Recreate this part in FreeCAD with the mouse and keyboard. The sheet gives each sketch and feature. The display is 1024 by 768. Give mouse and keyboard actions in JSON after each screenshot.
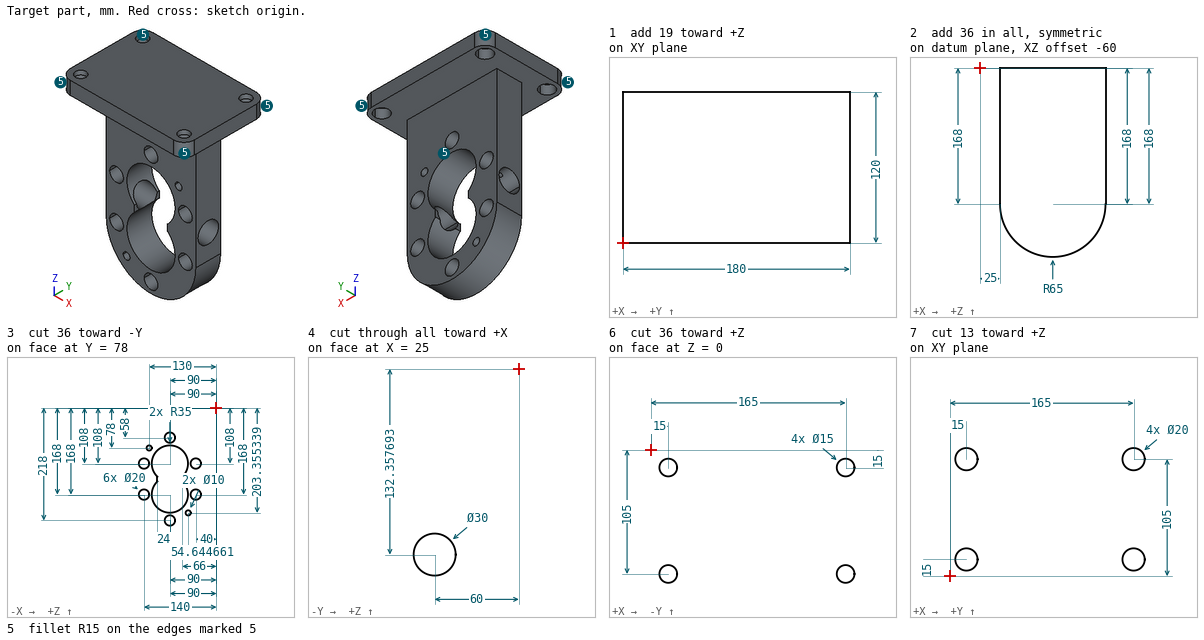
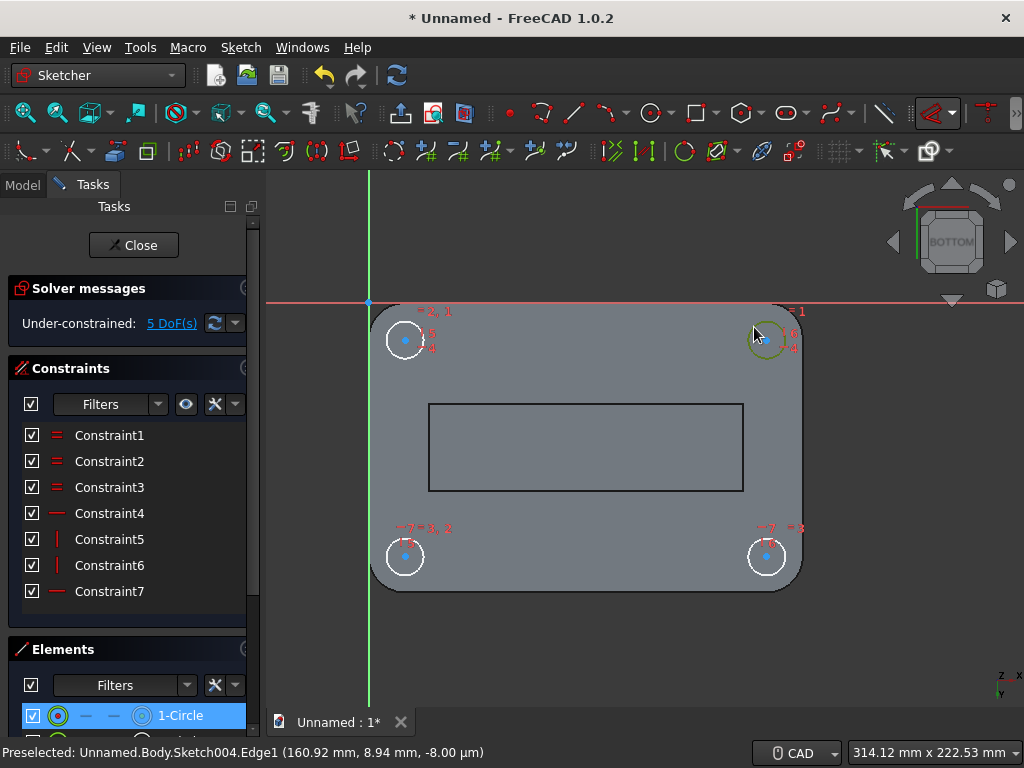
{"action": "left_click", "coordinate": [954, 114]}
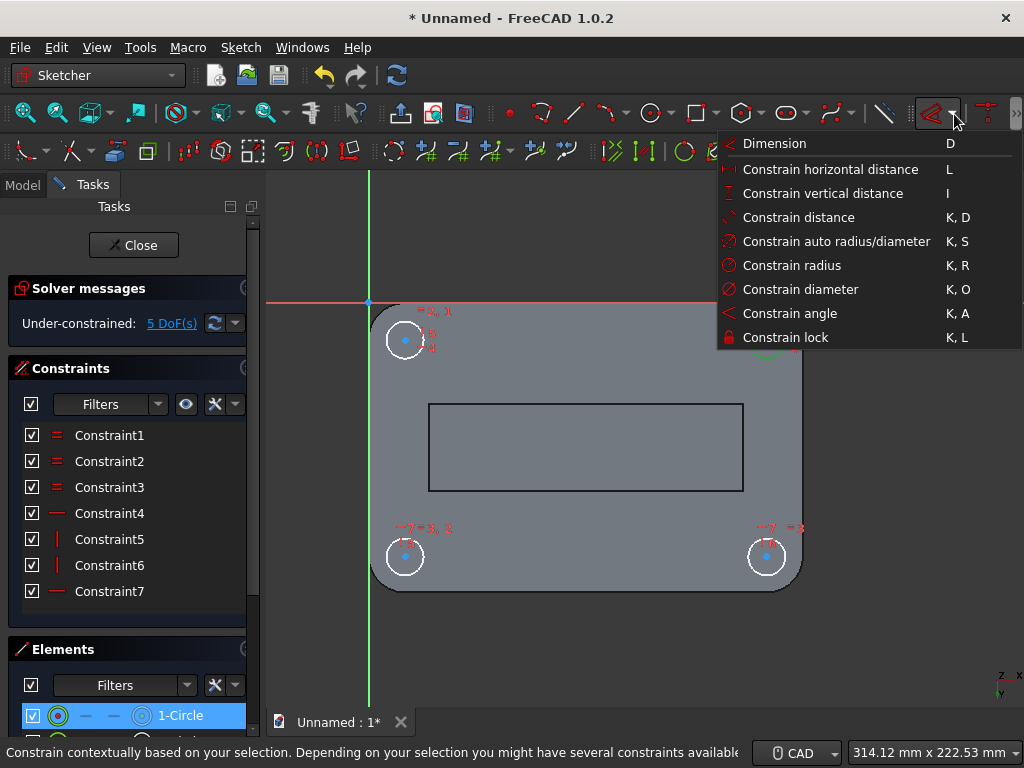
{"action": "left_click", "coordinate": [870, 289]}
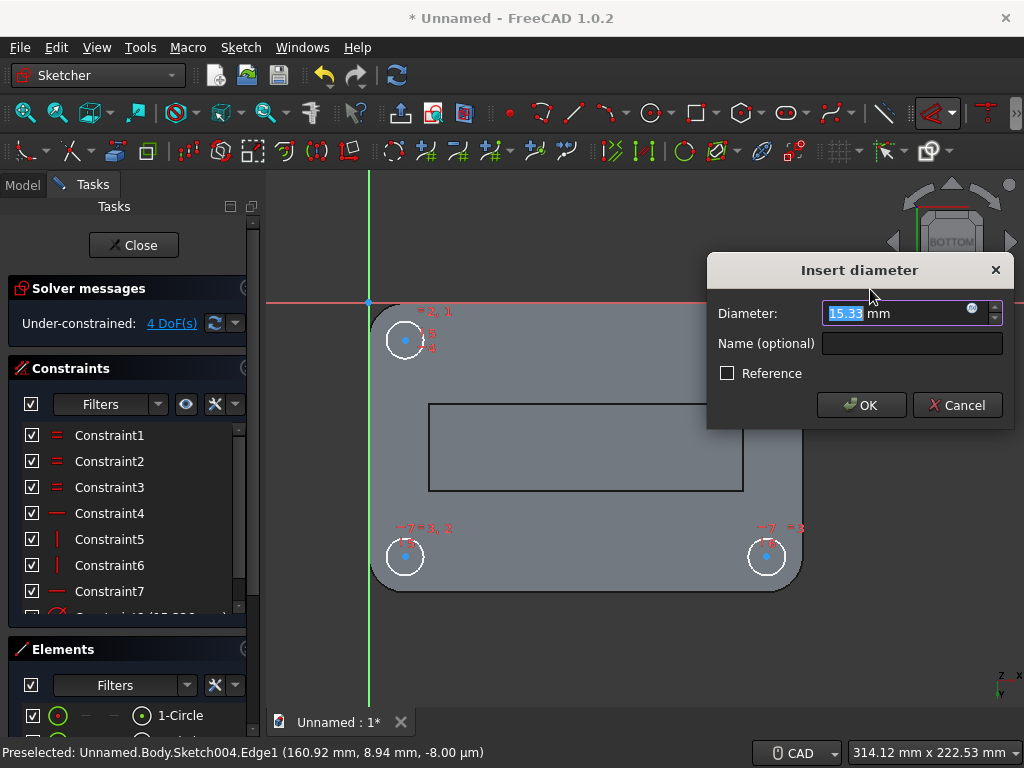
{"action": "type", "text": "15"}
{"action": "key", "text": "Return"}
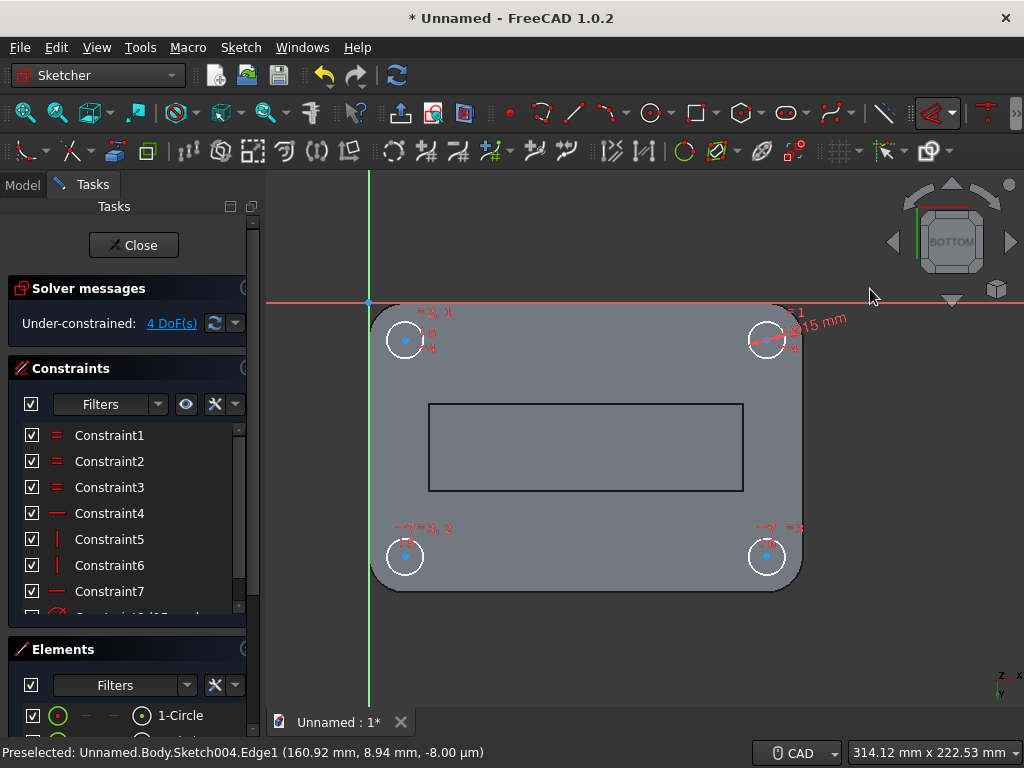
{"action": "left_click", "coordinate": [767, 340]}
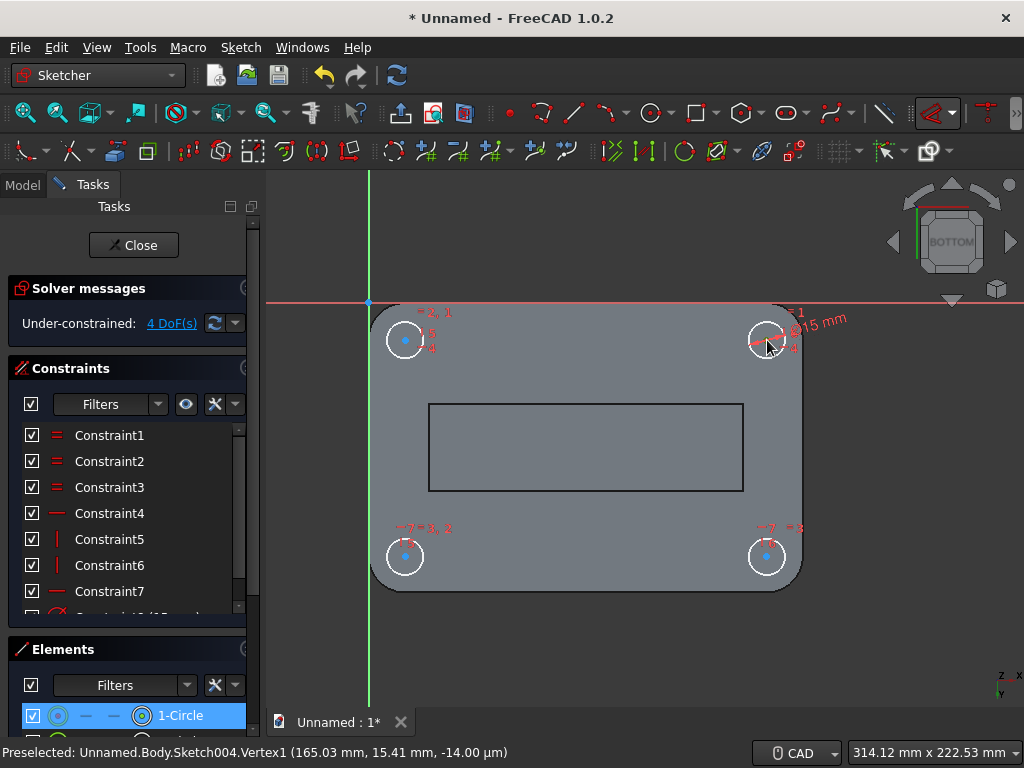
{"action": "left_click", "coordinate": [954, 114]}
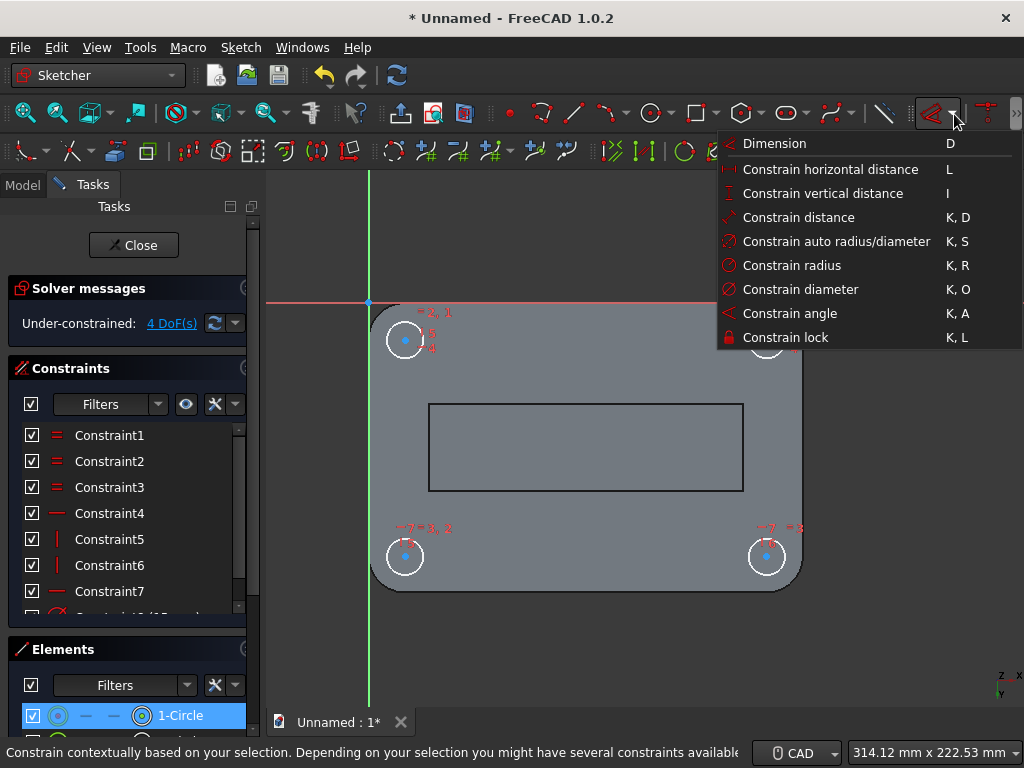
{"action": "left_click", "coordinate": [870, 193]}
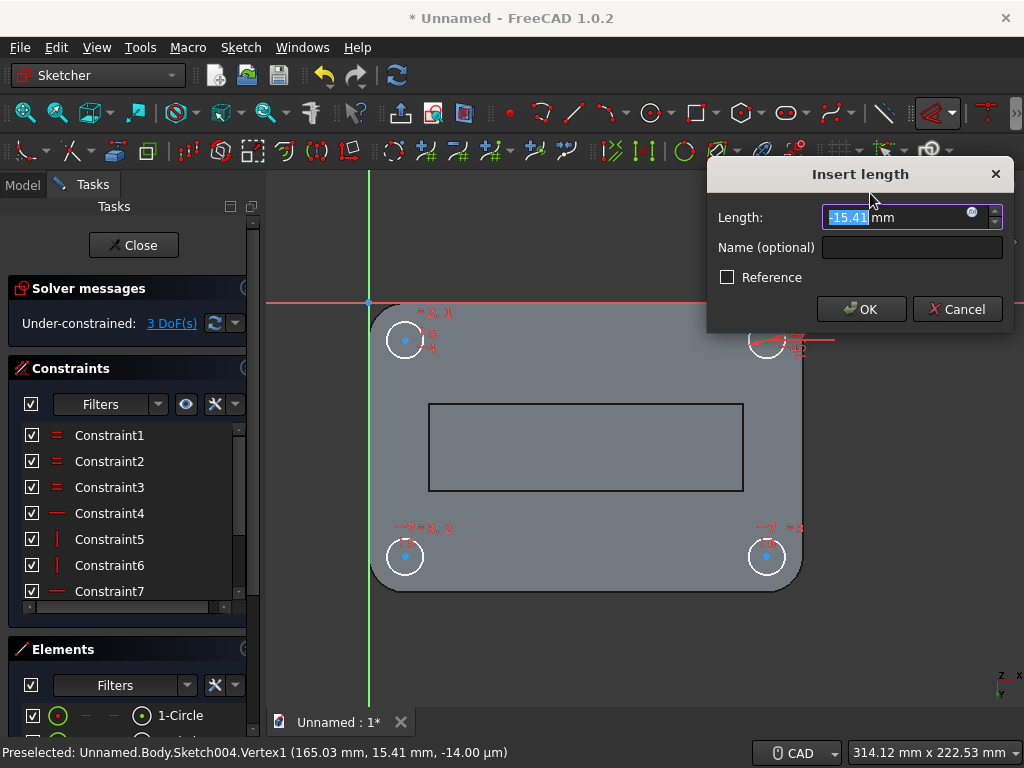
{"action": "type", "text": "-15"}
{"action": "key", "text": "Return"}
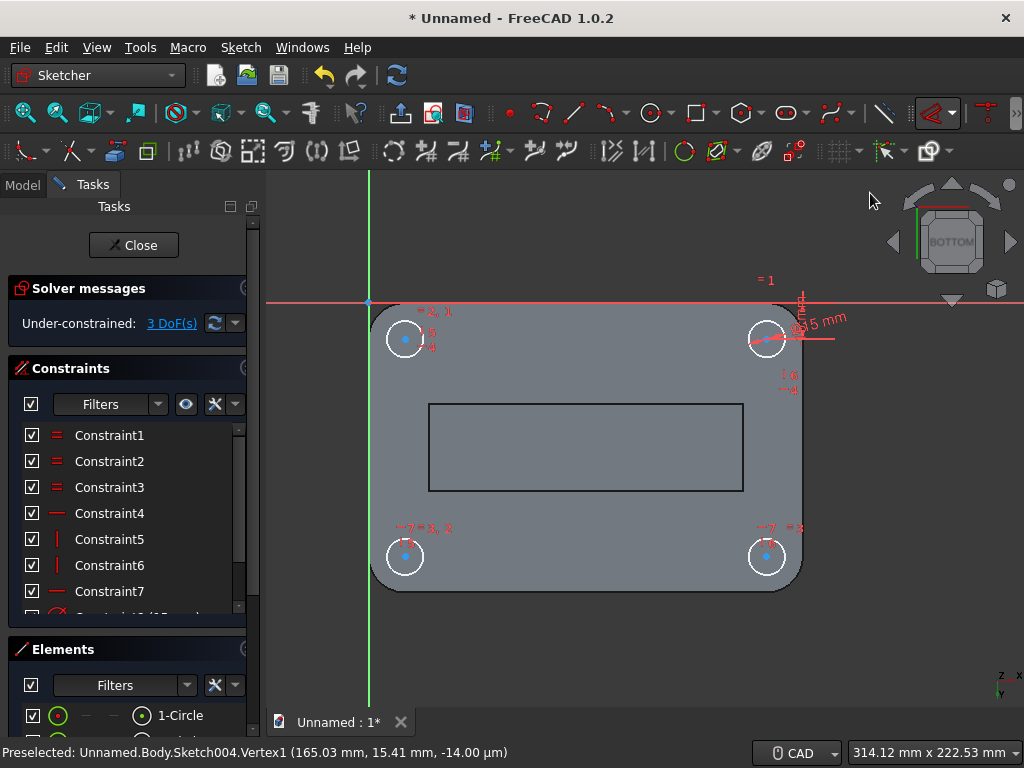
{"action": "left_click", "coordinate": [405, 339]}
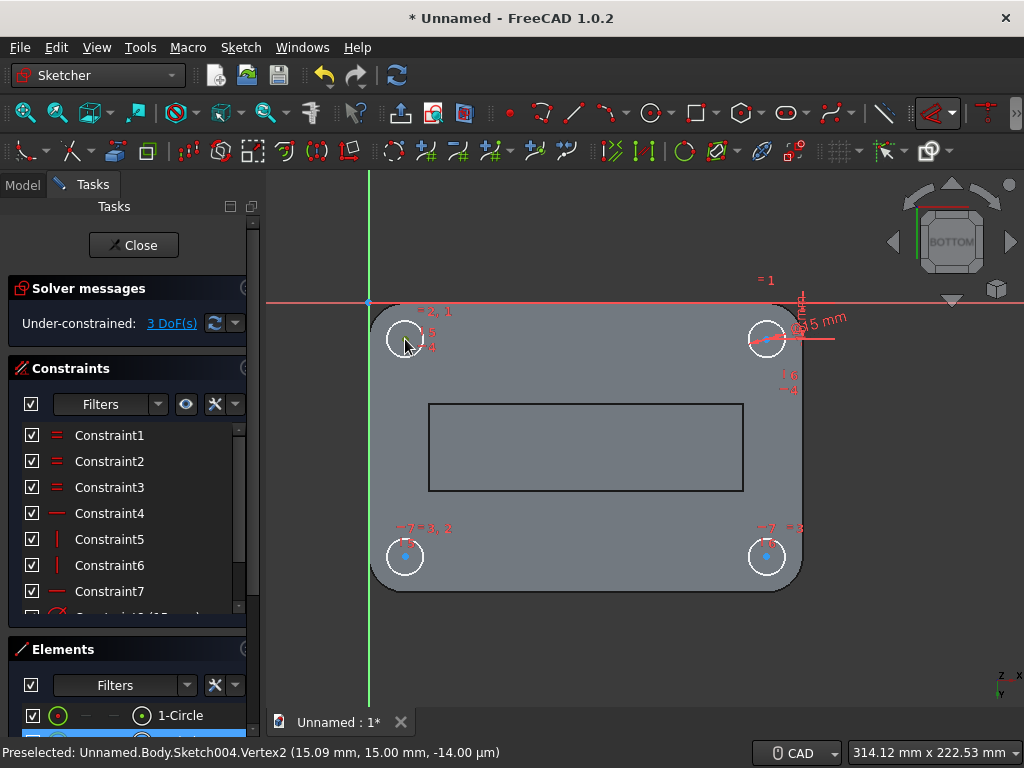
{"action": "left_click", "coordinate": [954, 114]}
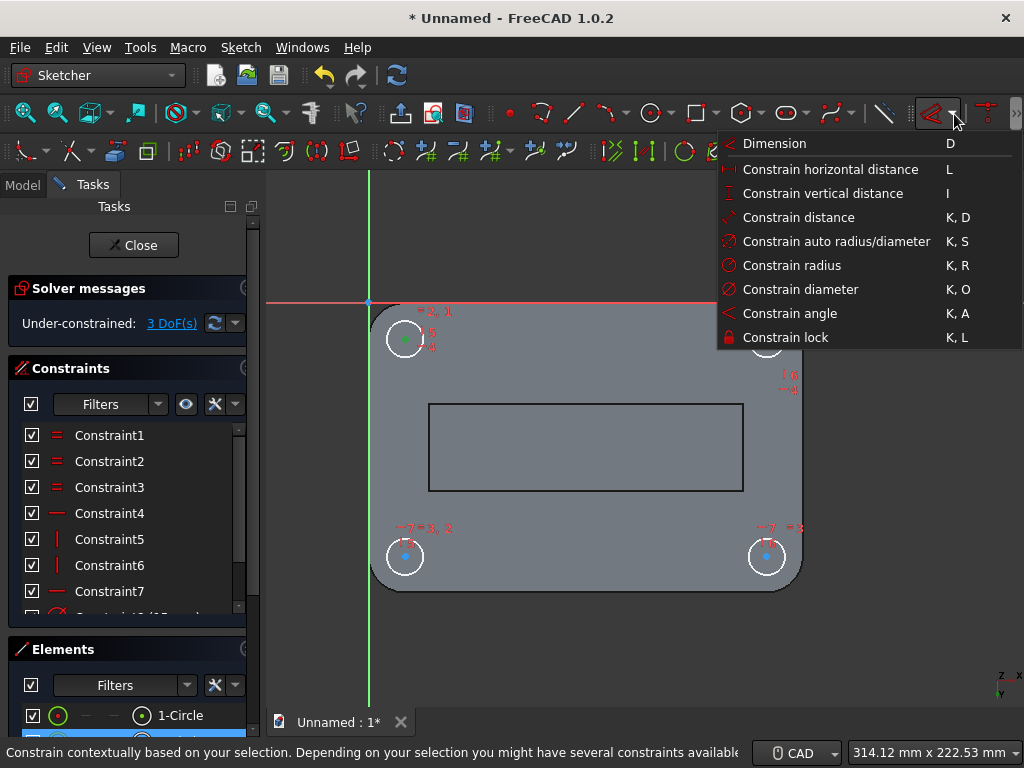
{"action": "left_click", "coordinate": [870, 169]}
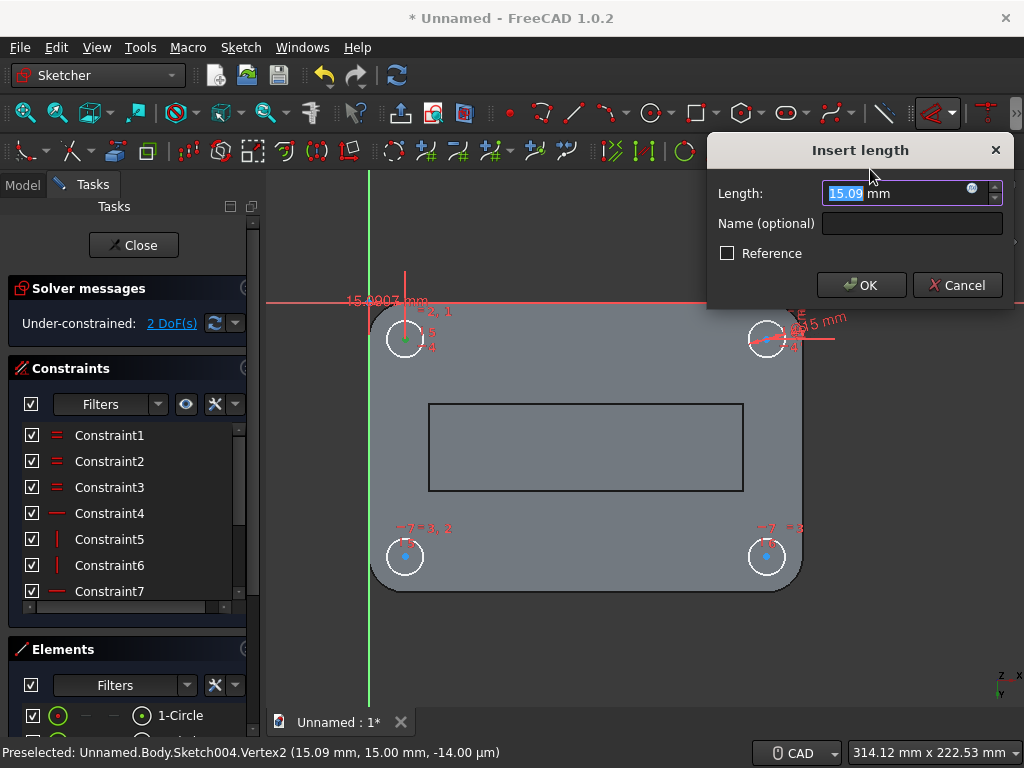
{"action": "type", "text": "15"}
{"action": "key", "text": "Return"}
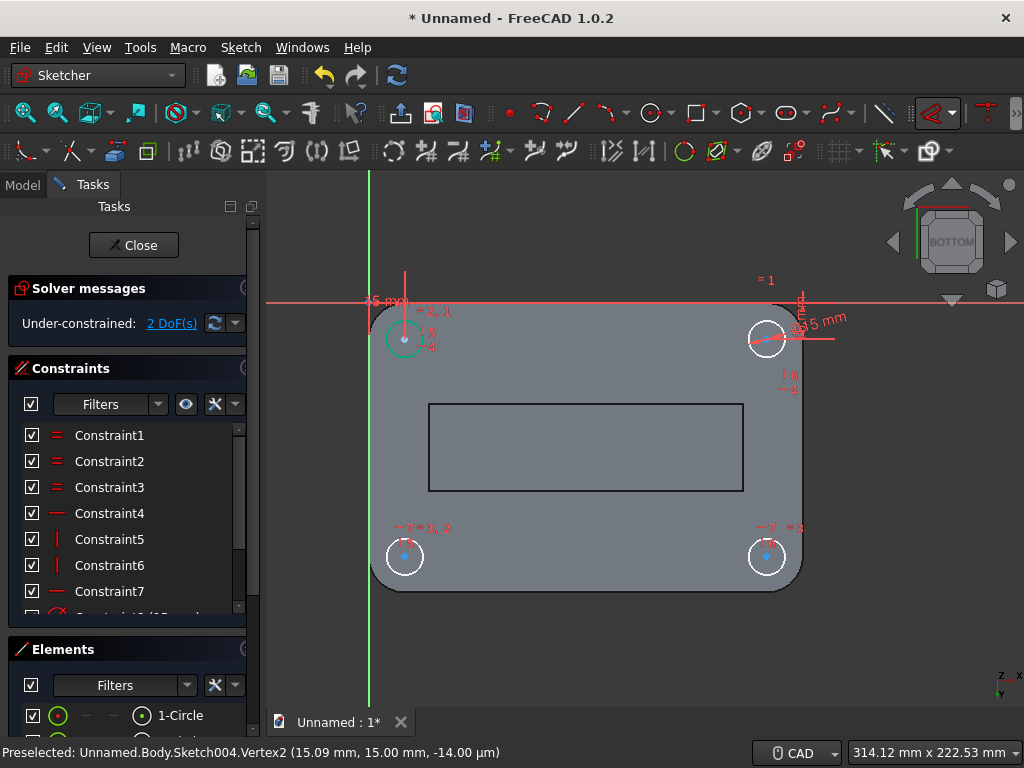
{"action": "left_click", "coordinate": [767, 339]}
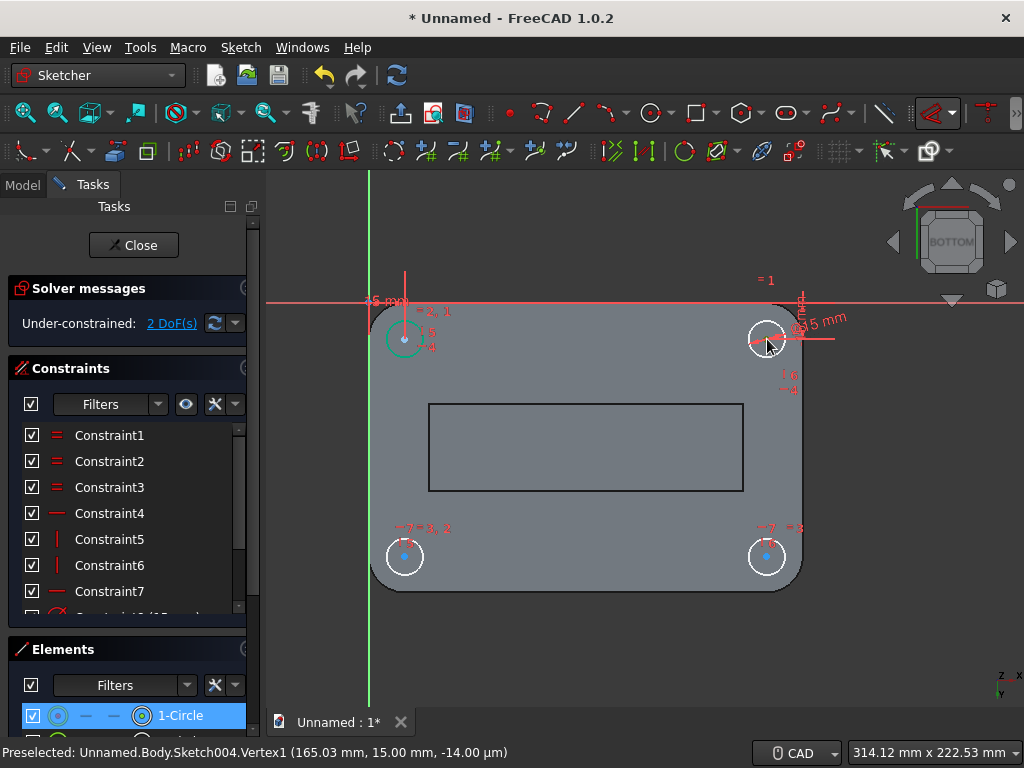
{"action": "key", "text": "l"}